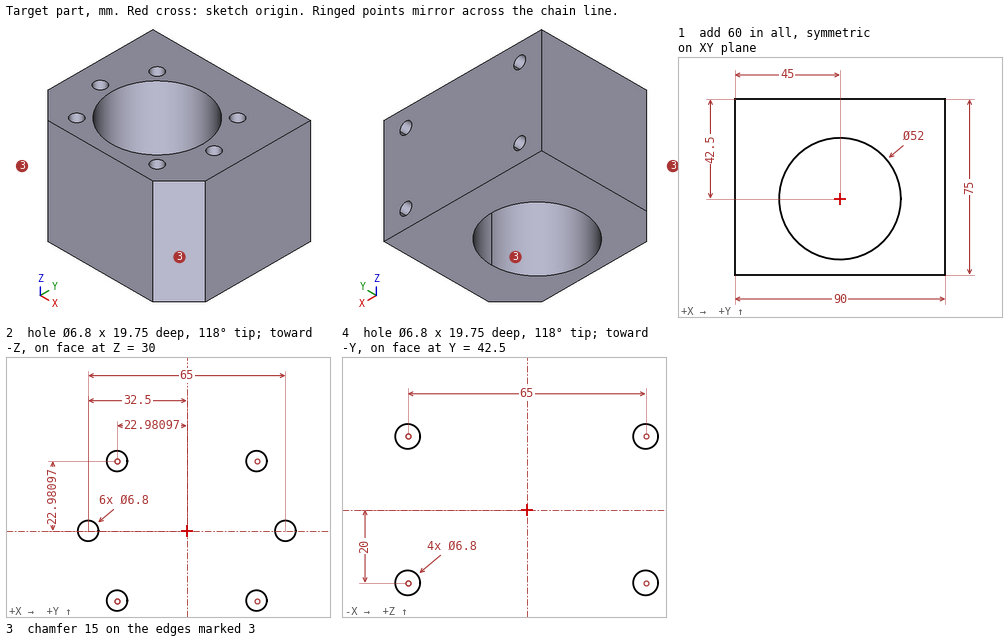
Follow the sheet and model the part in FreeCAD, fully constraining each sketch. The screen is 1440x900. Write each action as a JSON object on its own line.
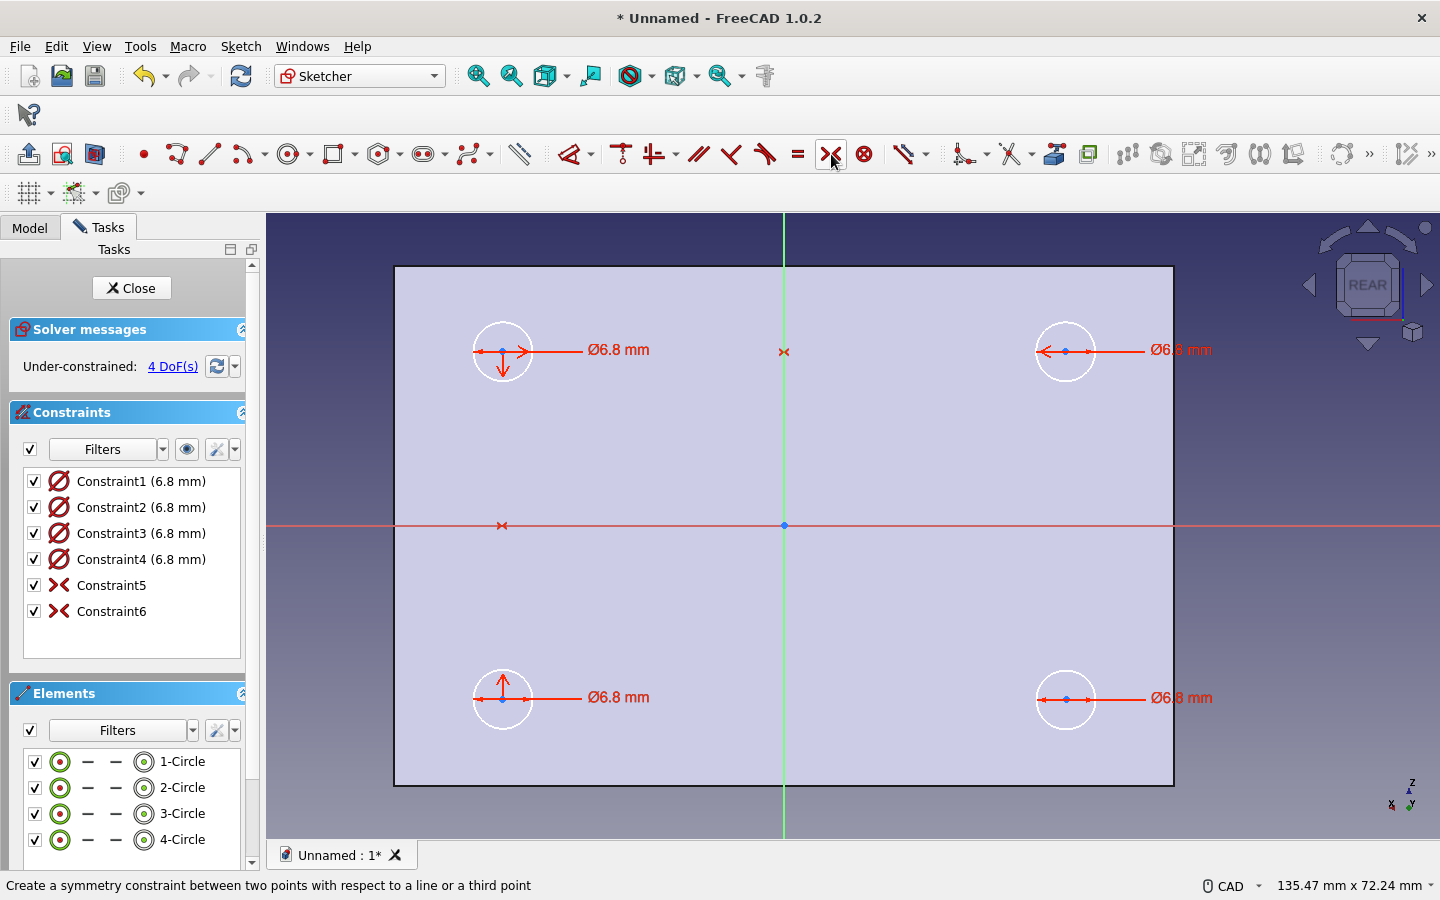
{"action": "left_click", "coordinate": [503, 699]}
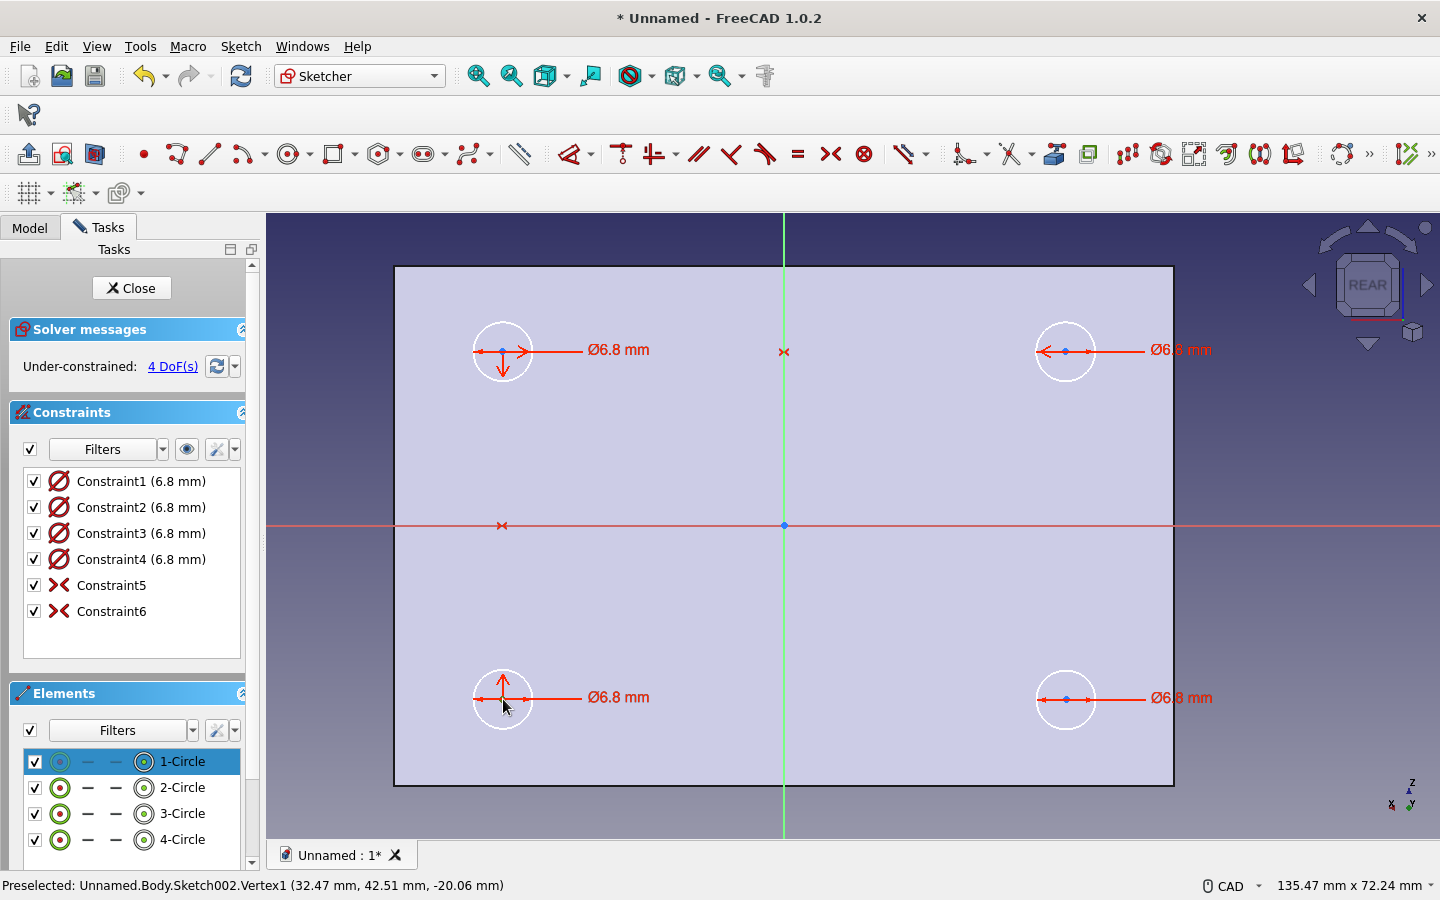
{"action": "left_click", "coordinate": [1066, 700]}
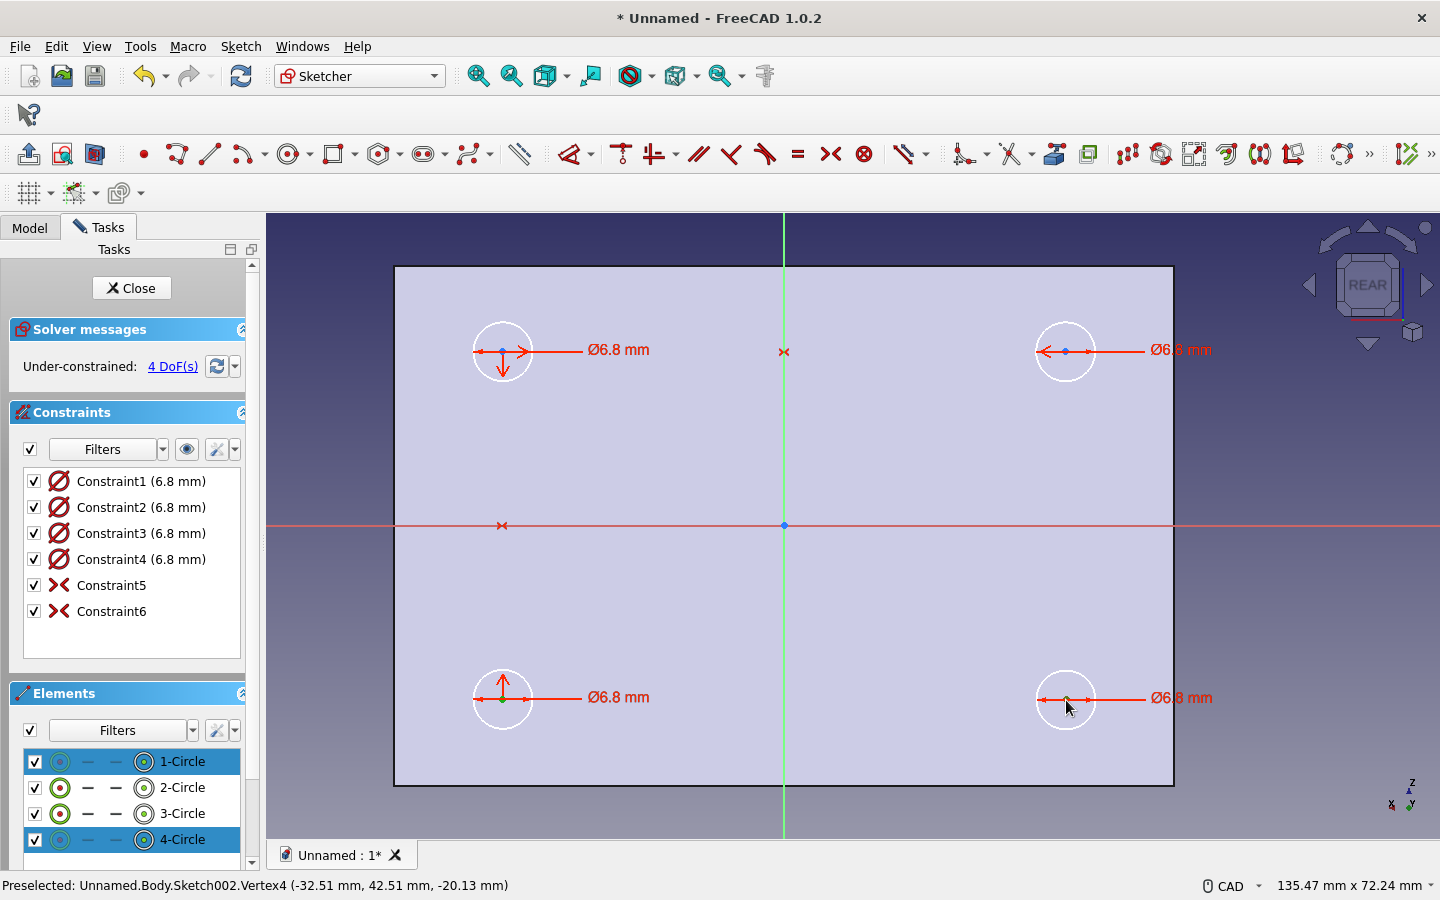
{"action": "left_click", "coordinate": [784, 770]}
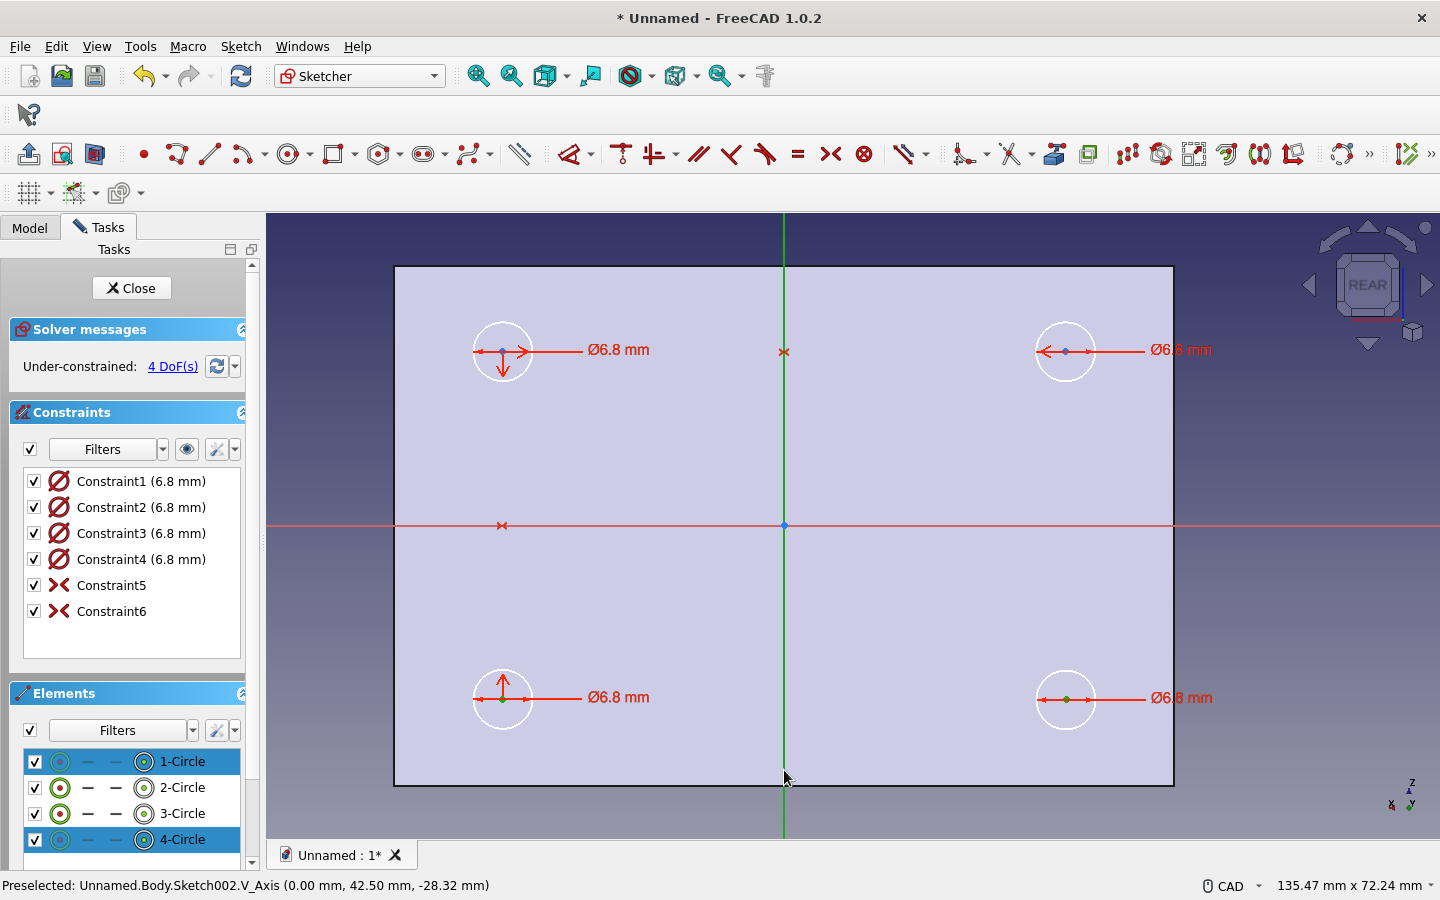
{"action": "left_click", "coordinate": [831, 154]}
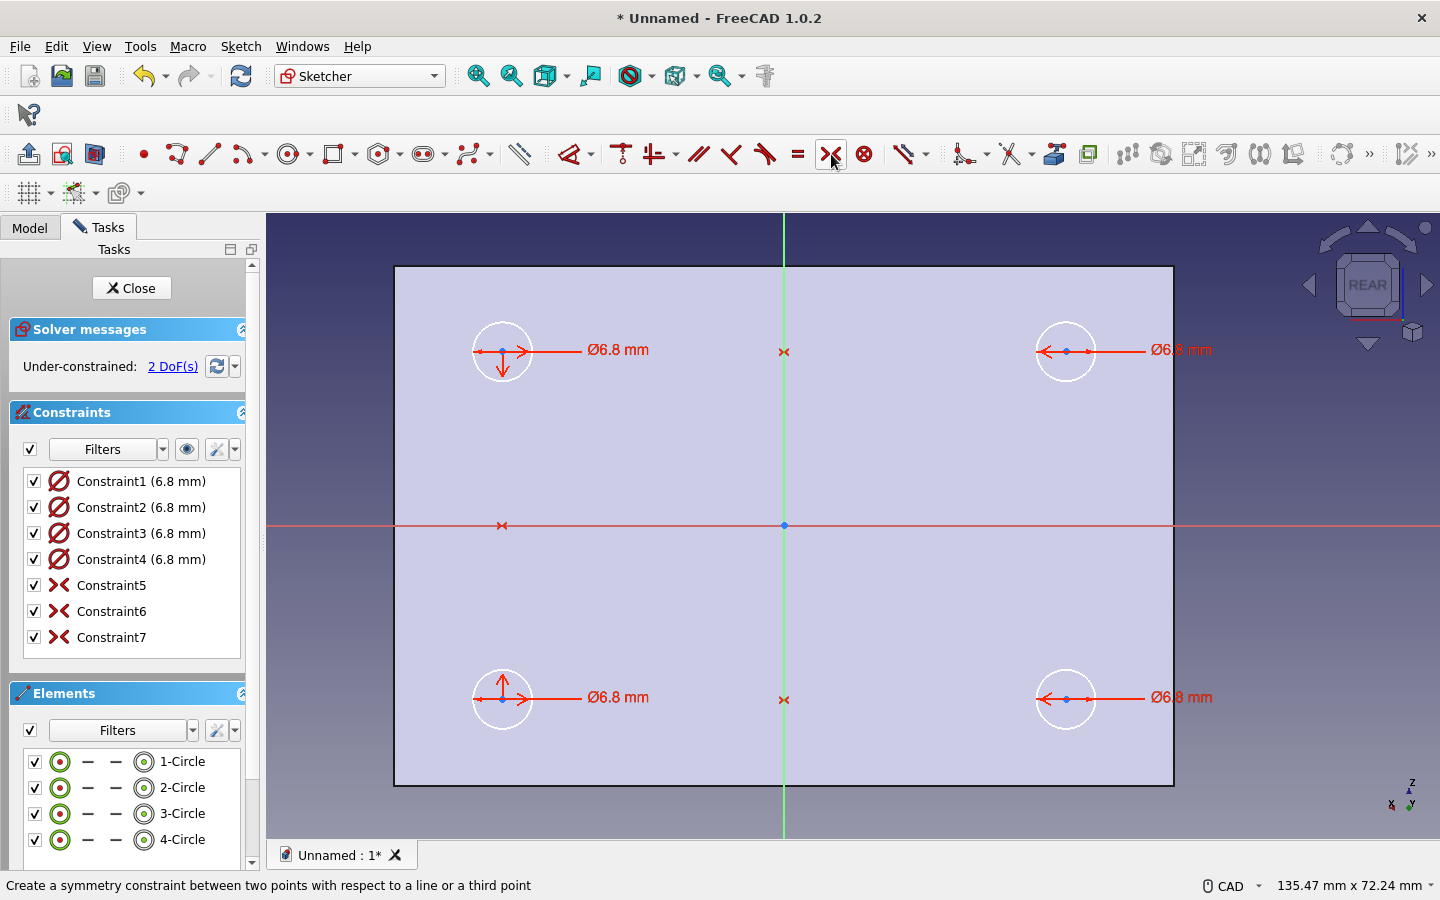
{"action": "left_click", "coordinate": [568, 154]}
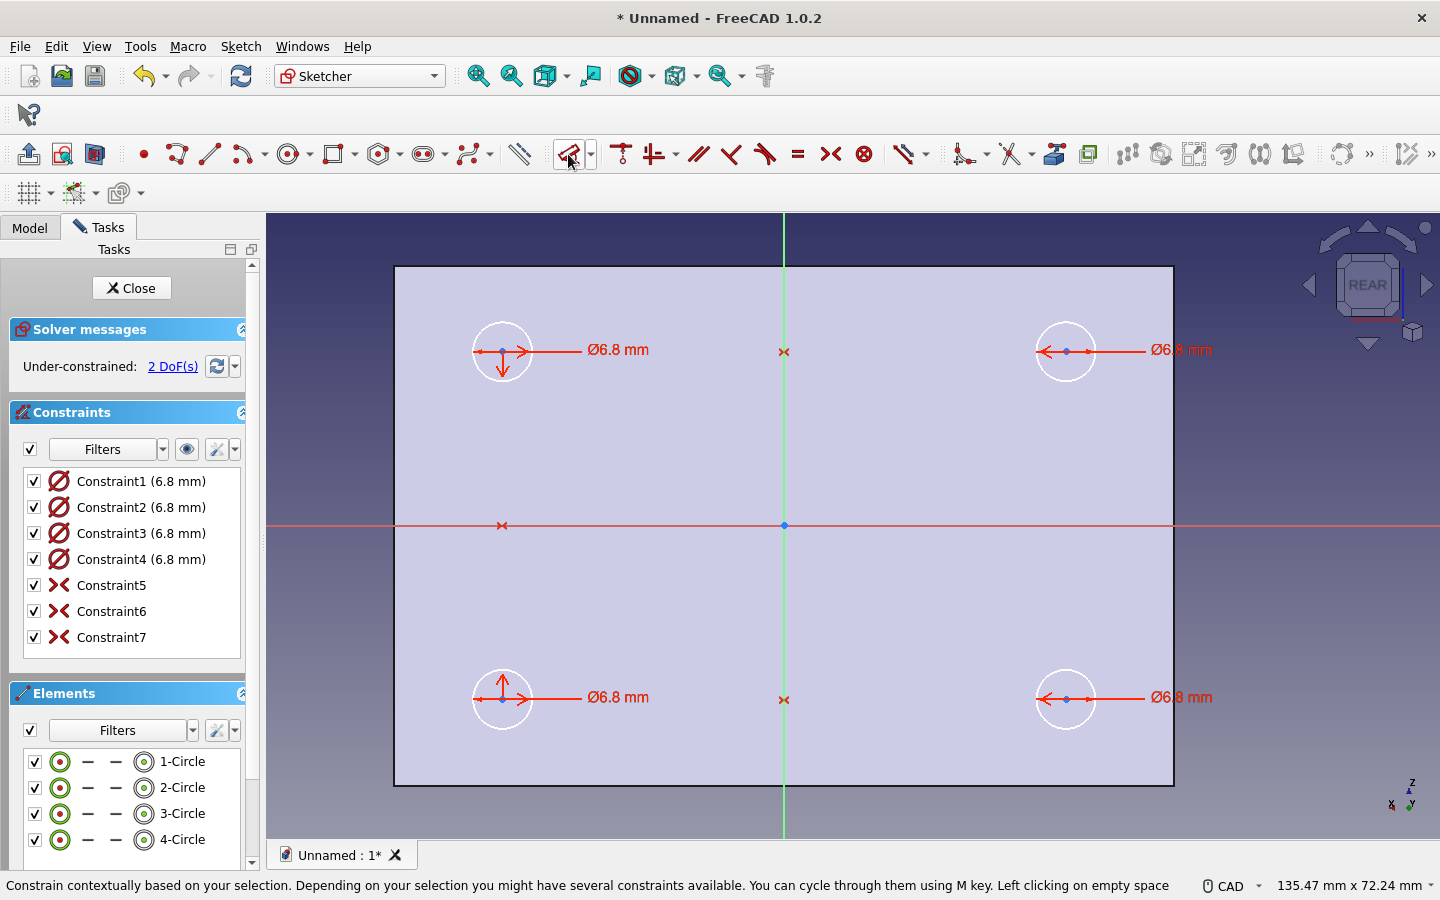
{"action": "left_click", "coordinate": [503, 699]}
{"action": "left_click", "coordinate": [469, 612]}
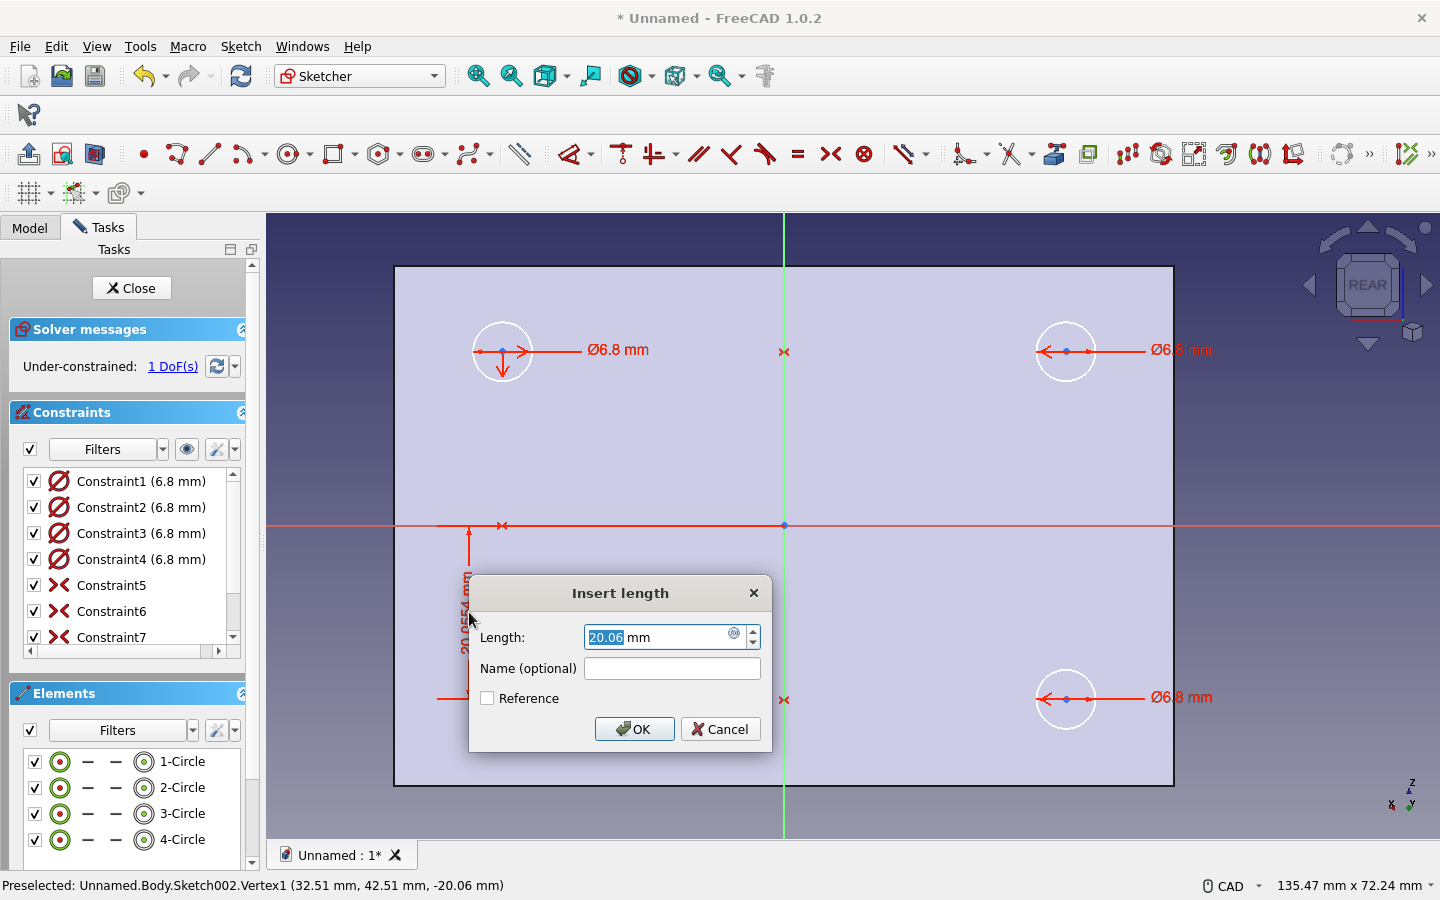
{"action": "type", "text": "20"}
{"action": "key", "text": "Return"}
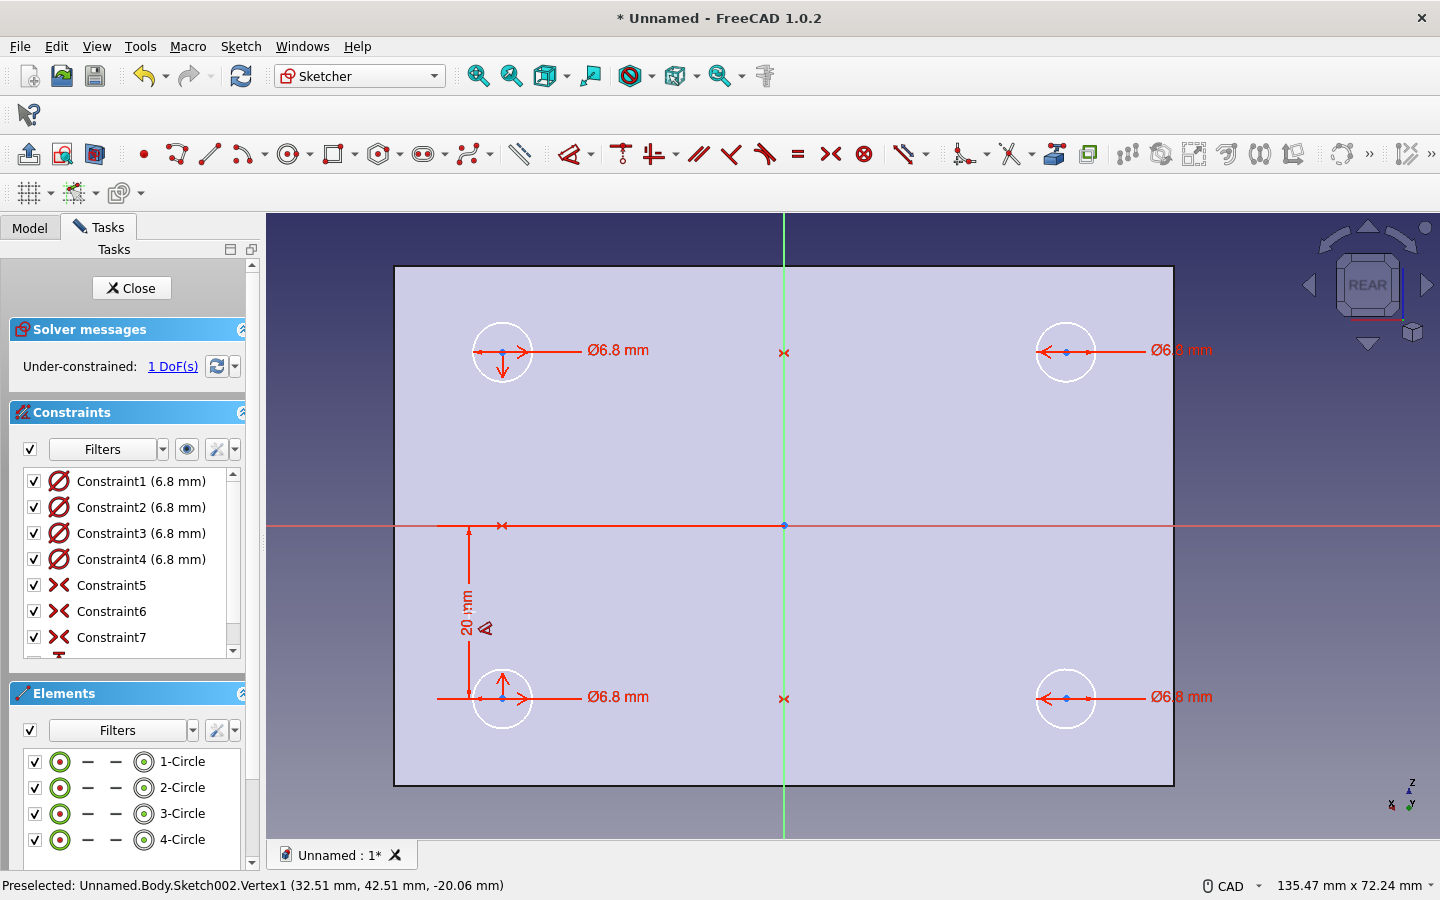
{"action": "left_click", "coordinate": [503, 352]}